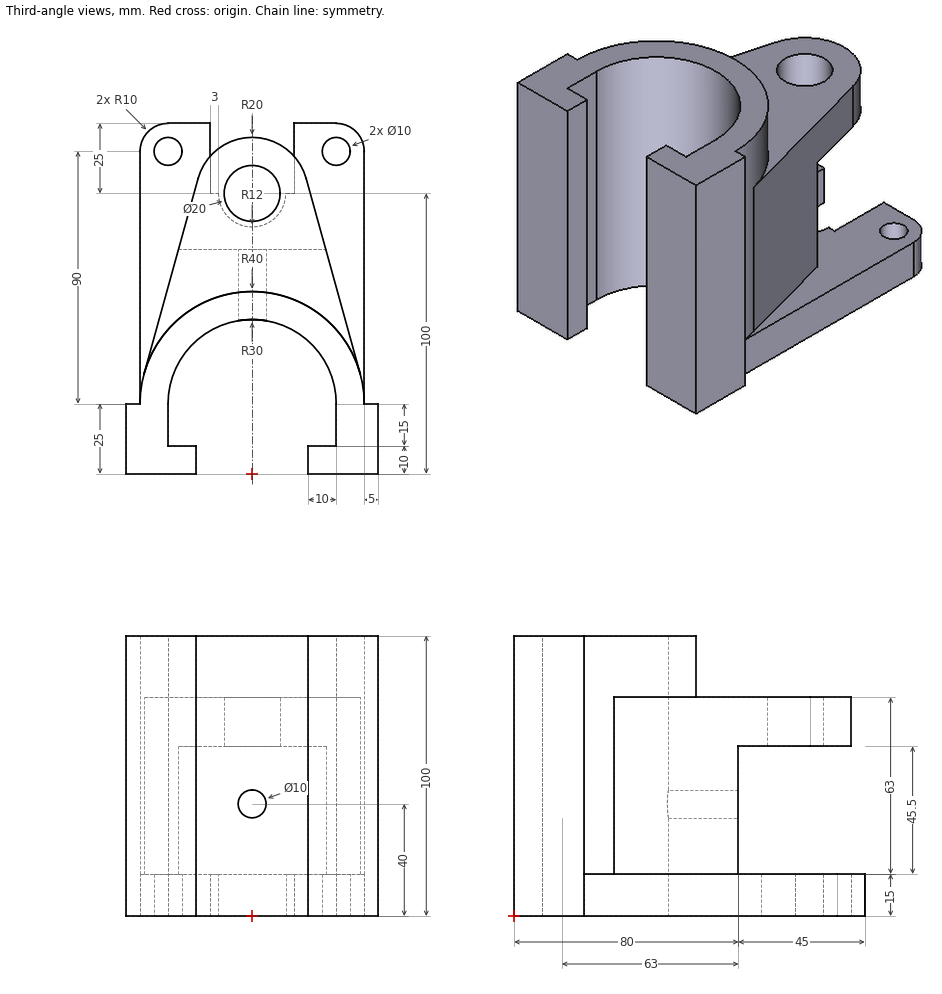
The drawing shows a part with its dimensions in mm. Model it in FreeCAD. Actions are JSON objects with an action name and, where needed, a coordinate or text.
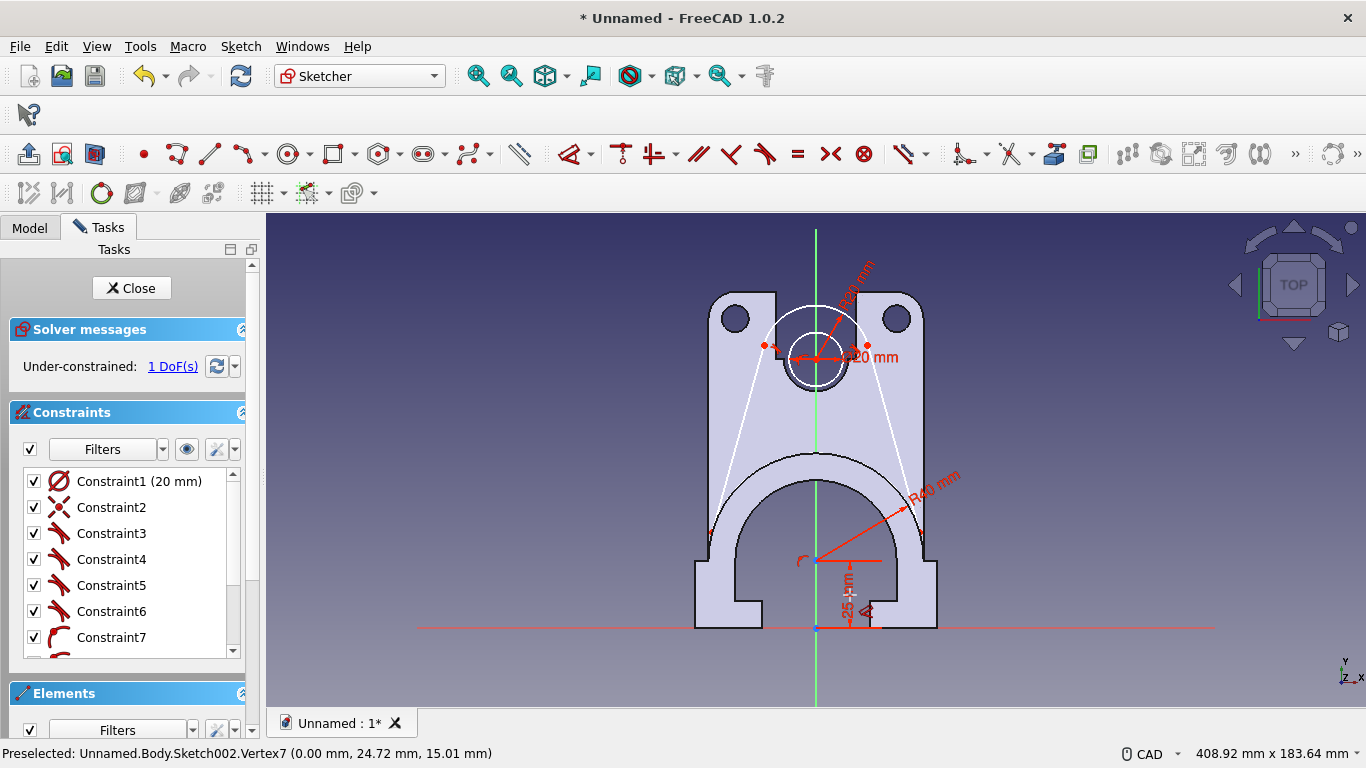
{"action": "left_click", "coordinate": [816, 359]}
{"action": "left_click", "coordinate": [850, 494]}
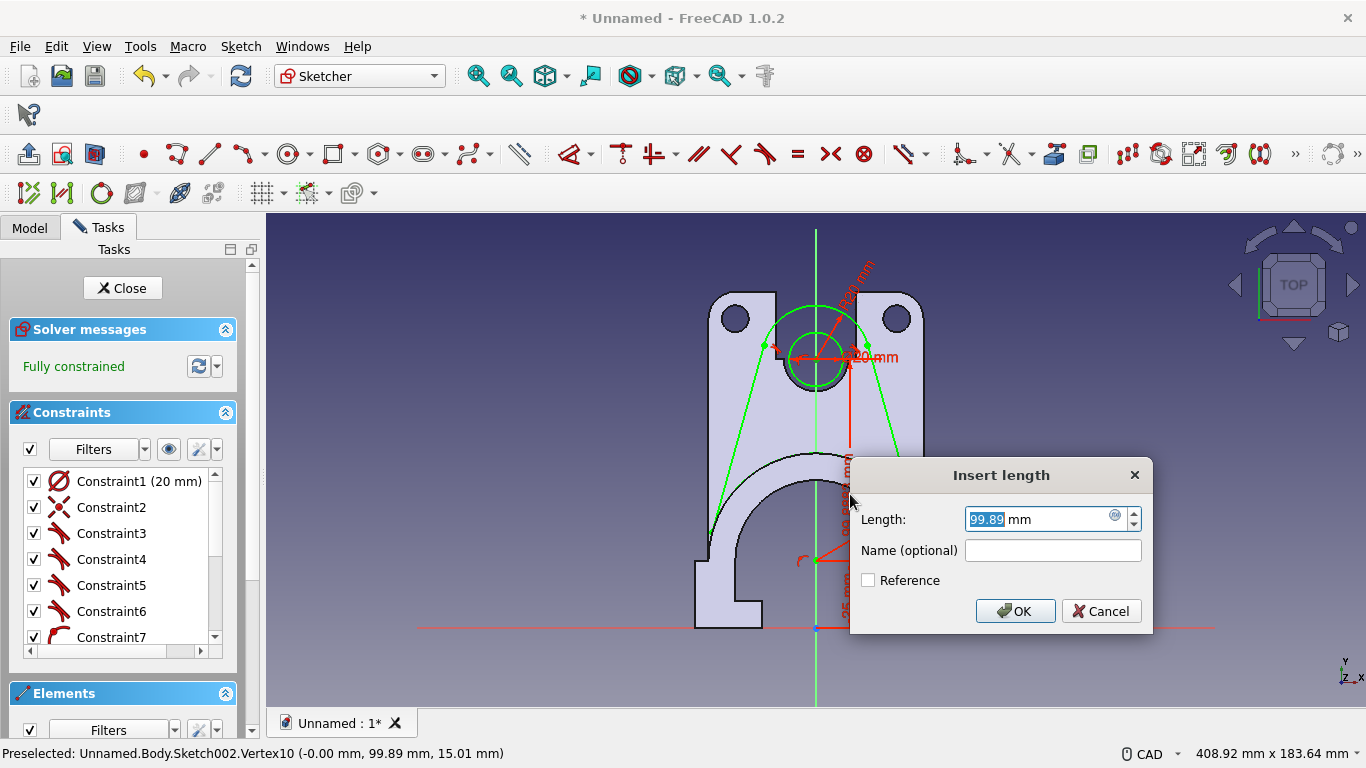
{"action": "type", "text": "100"}
{"action": "key", "text": "Return"}
{"action": "key", "text": "Escape"}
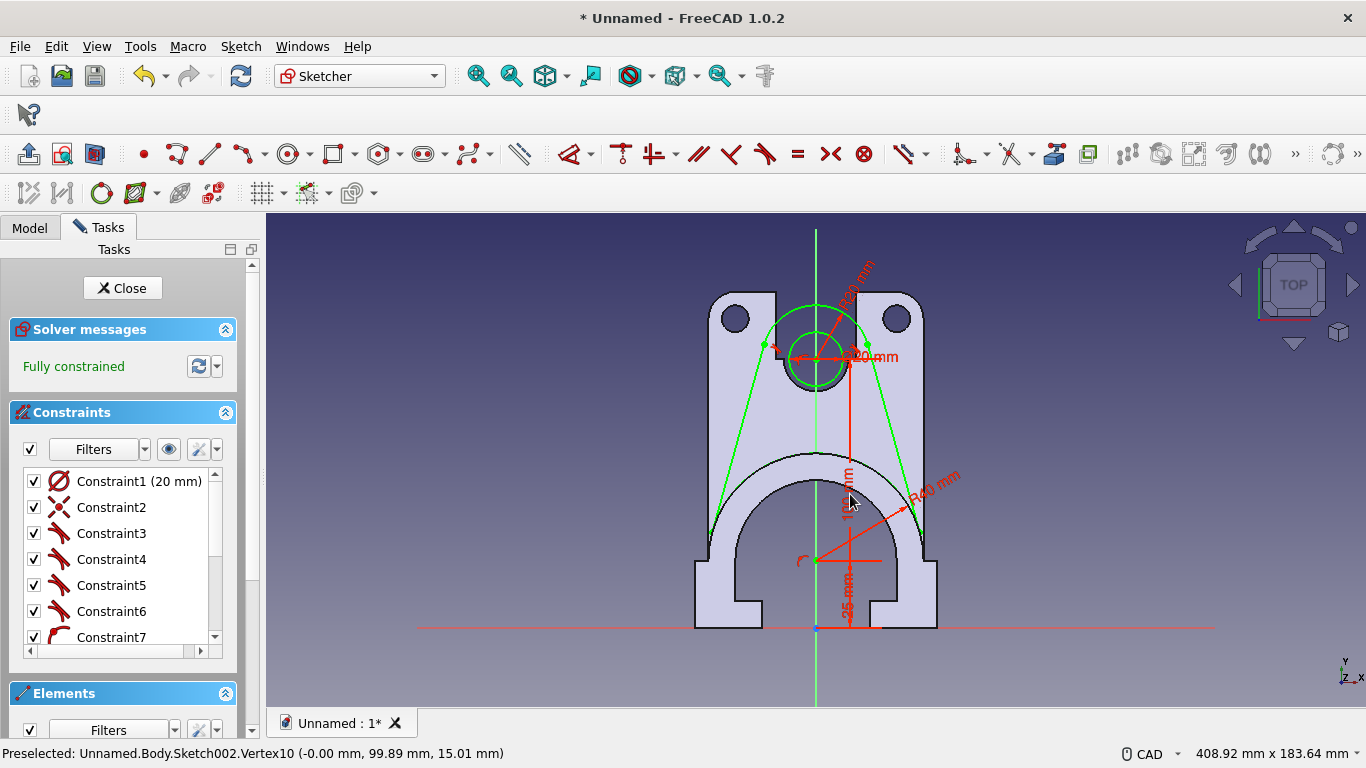
{"action": "left_click", "coordinate": [123, 288]}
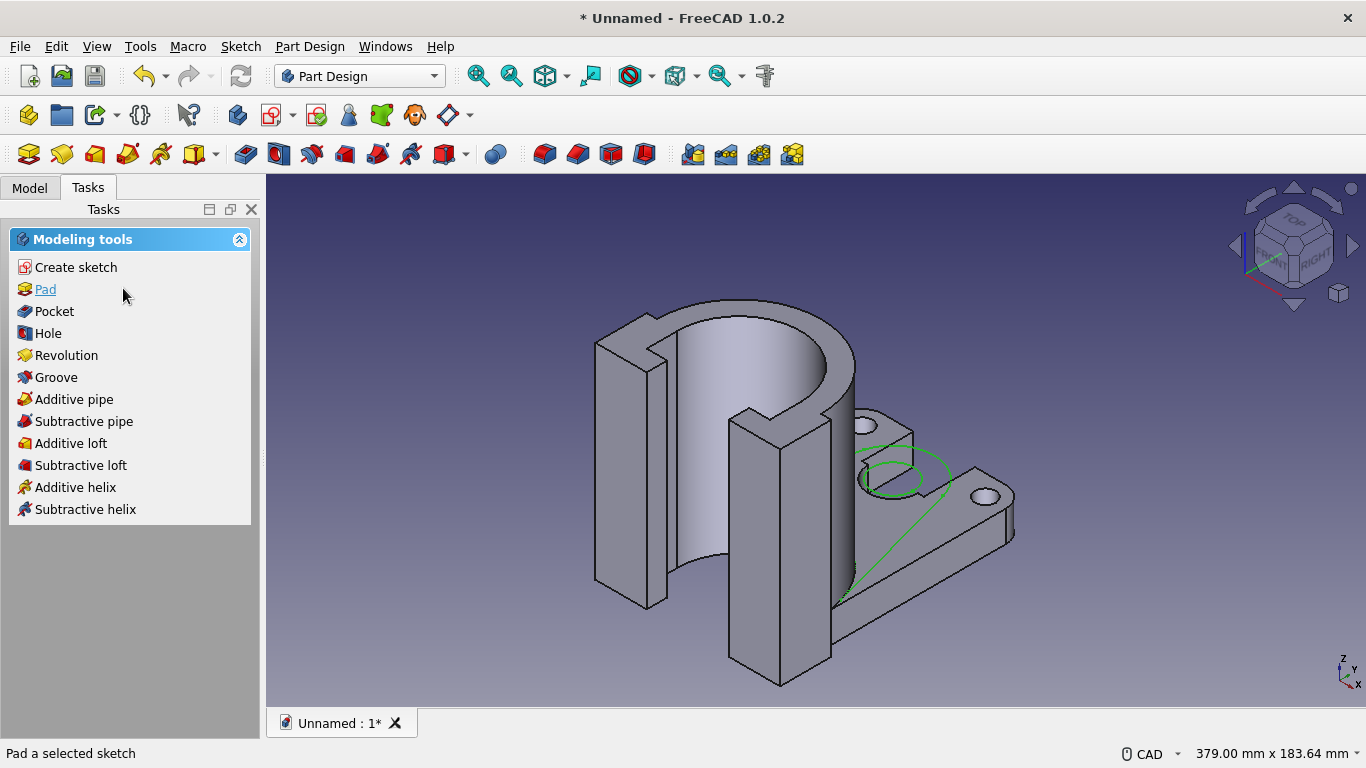
{"action": "left_click", "coordinate": [29, 154]}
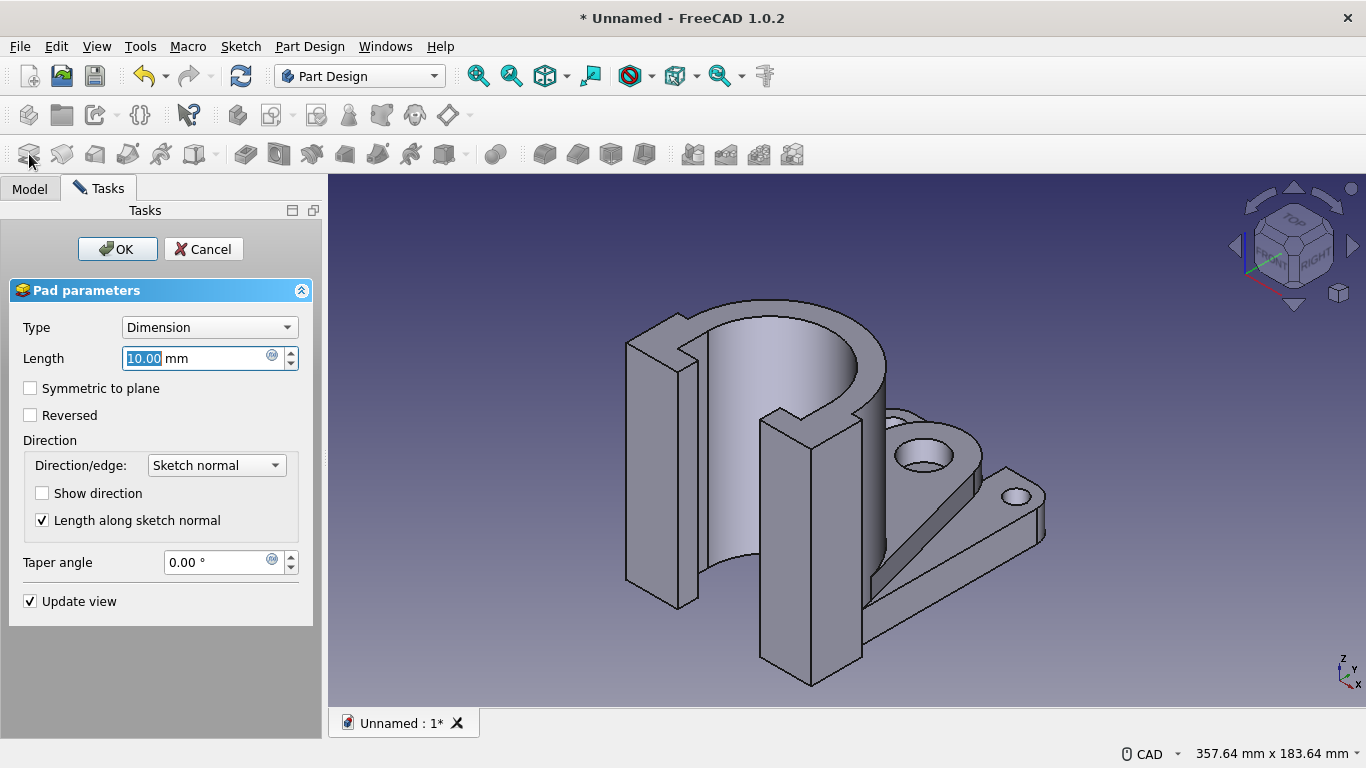
{"action": "type", "text": "63"}
{"action": "key", "text": "Tab"}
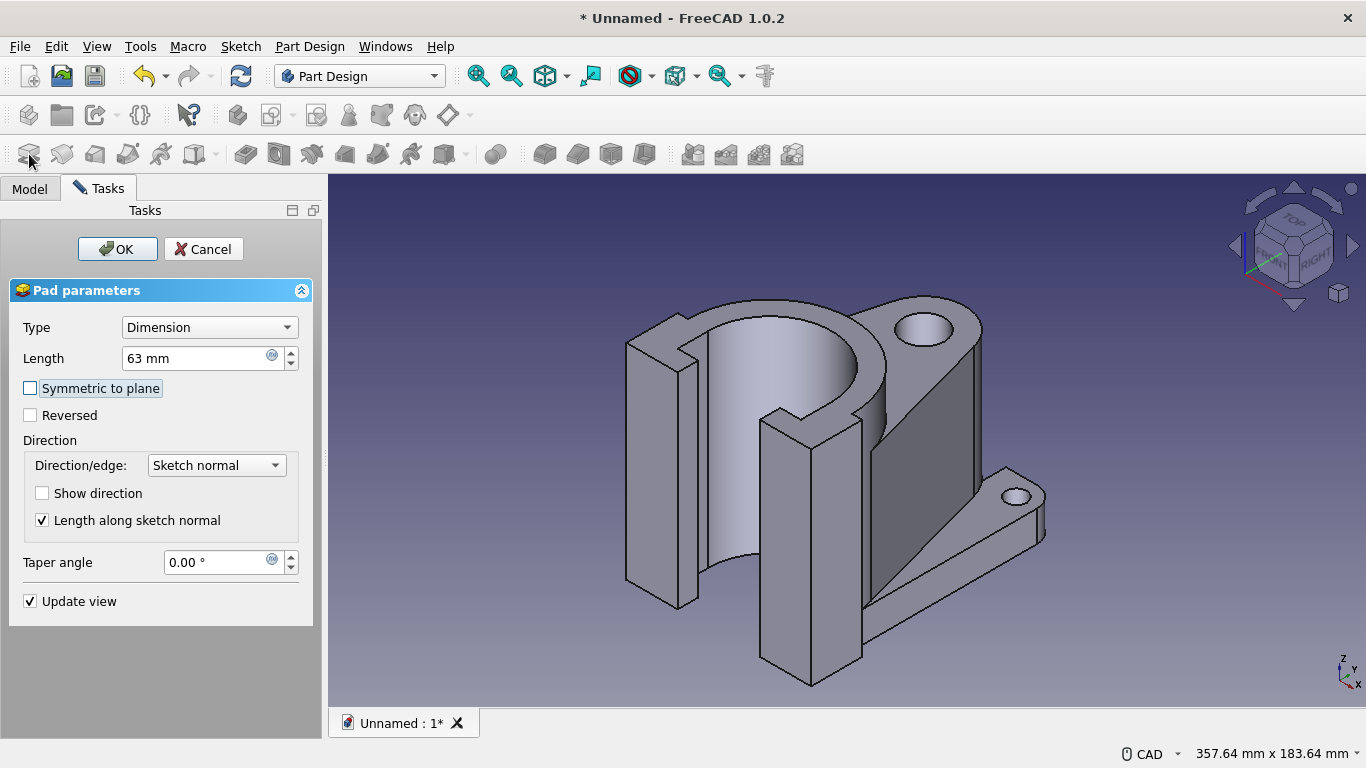
{"action": "left_click", "coordinate": [118, 249]}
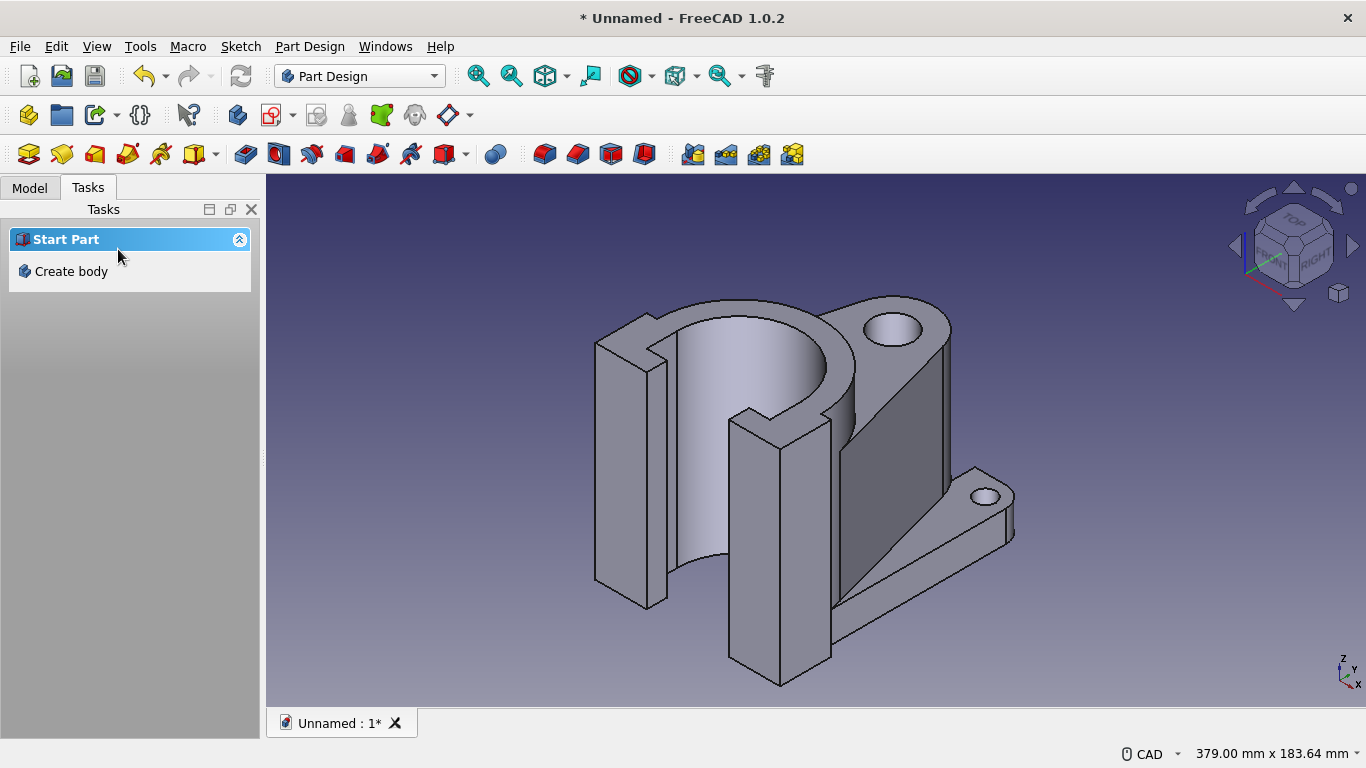
{"action": "left_click", "coordinate": [270, 116]}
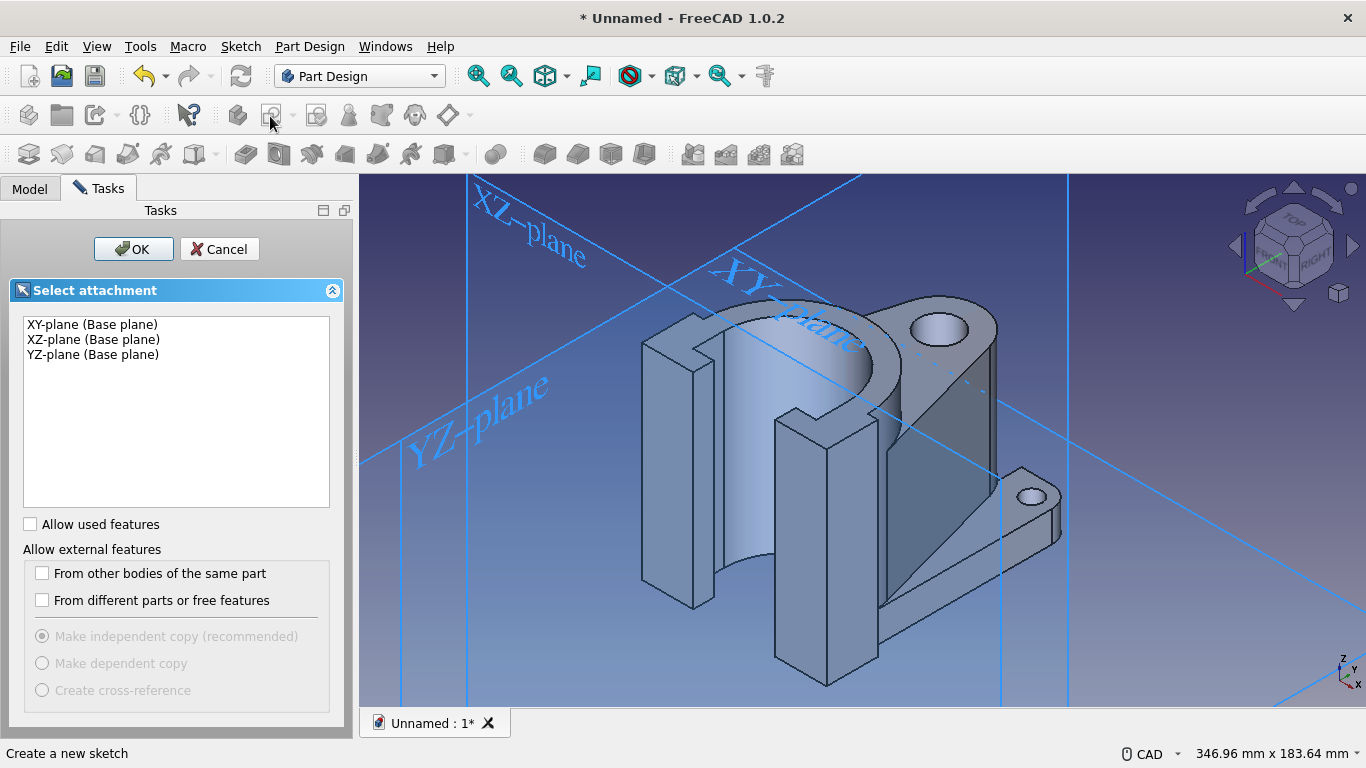
{"action": "left_click", "coordinate": [84, 354]}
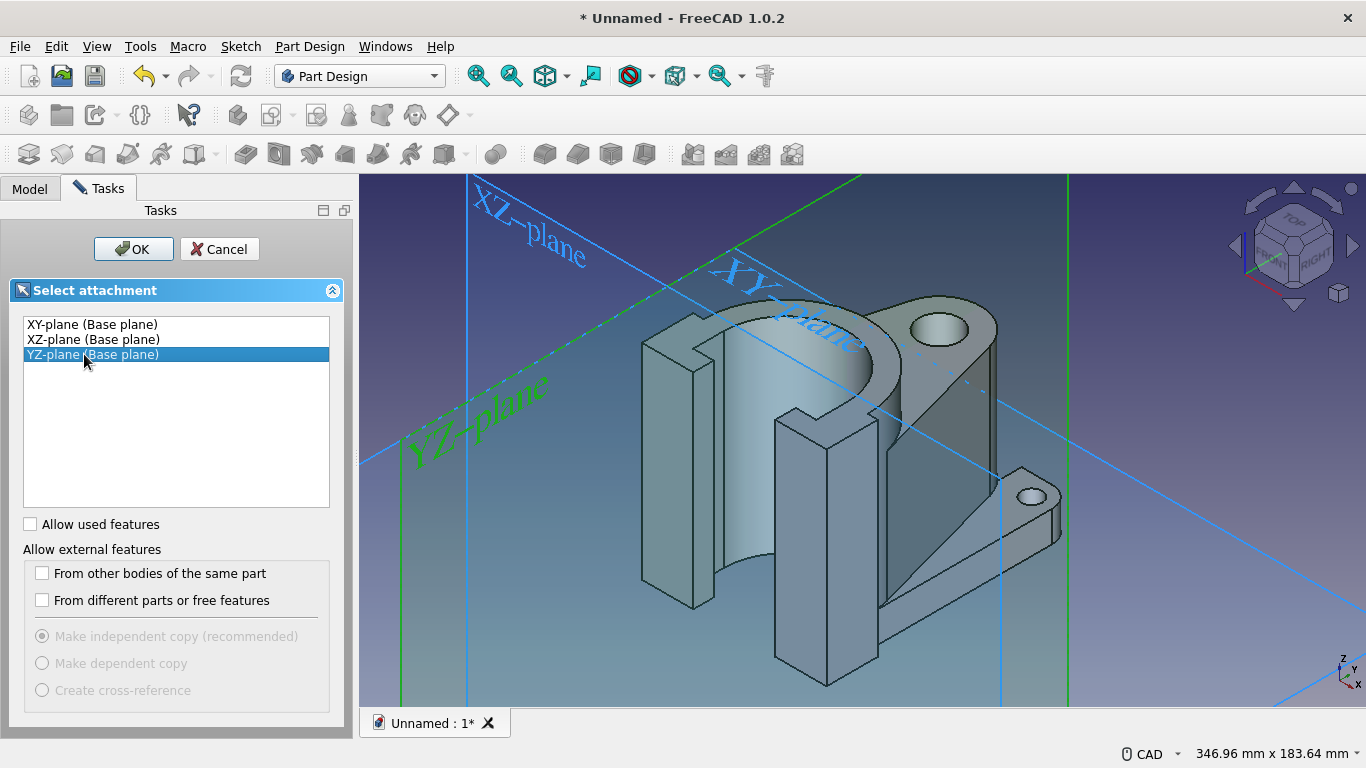
{"action": "left_click", "coordinate": [134, 249]}